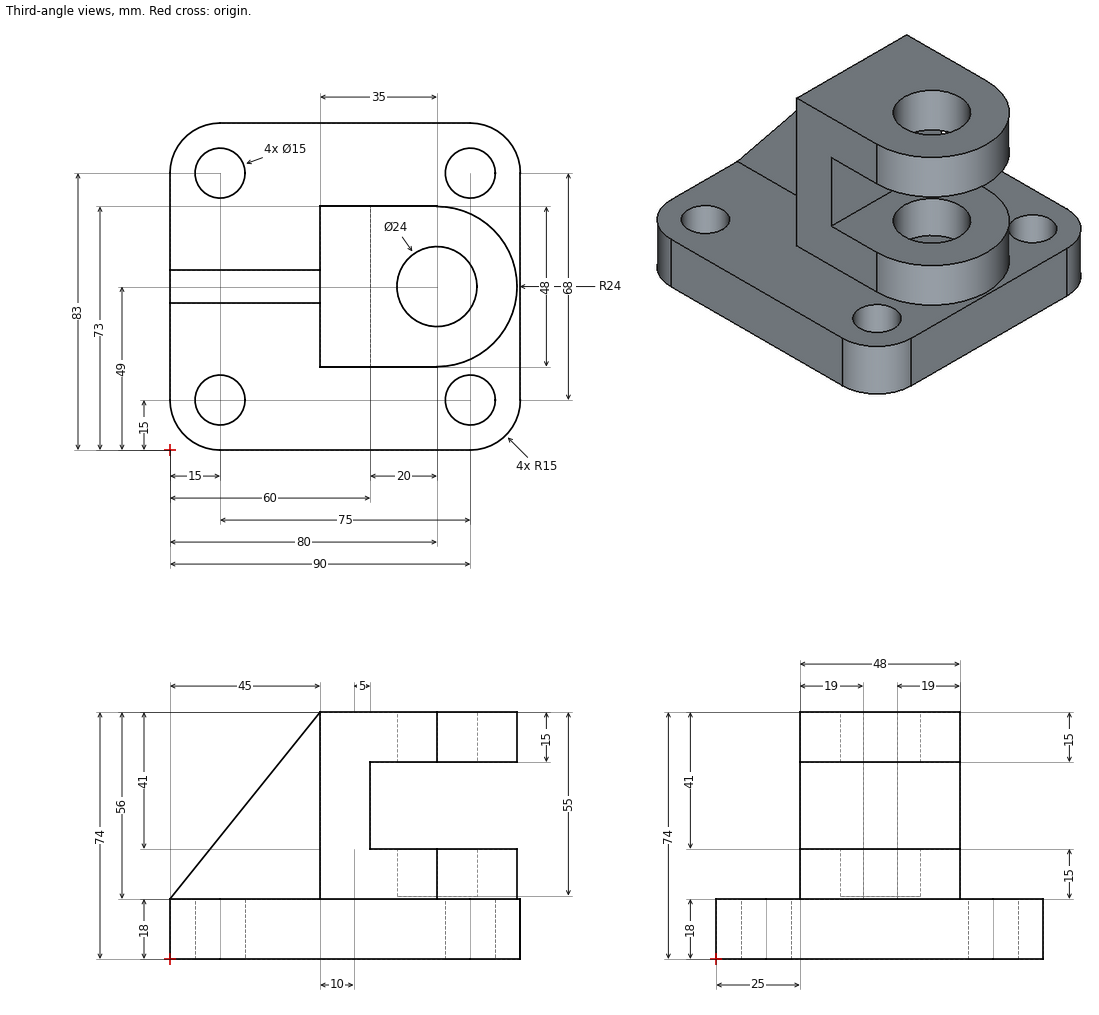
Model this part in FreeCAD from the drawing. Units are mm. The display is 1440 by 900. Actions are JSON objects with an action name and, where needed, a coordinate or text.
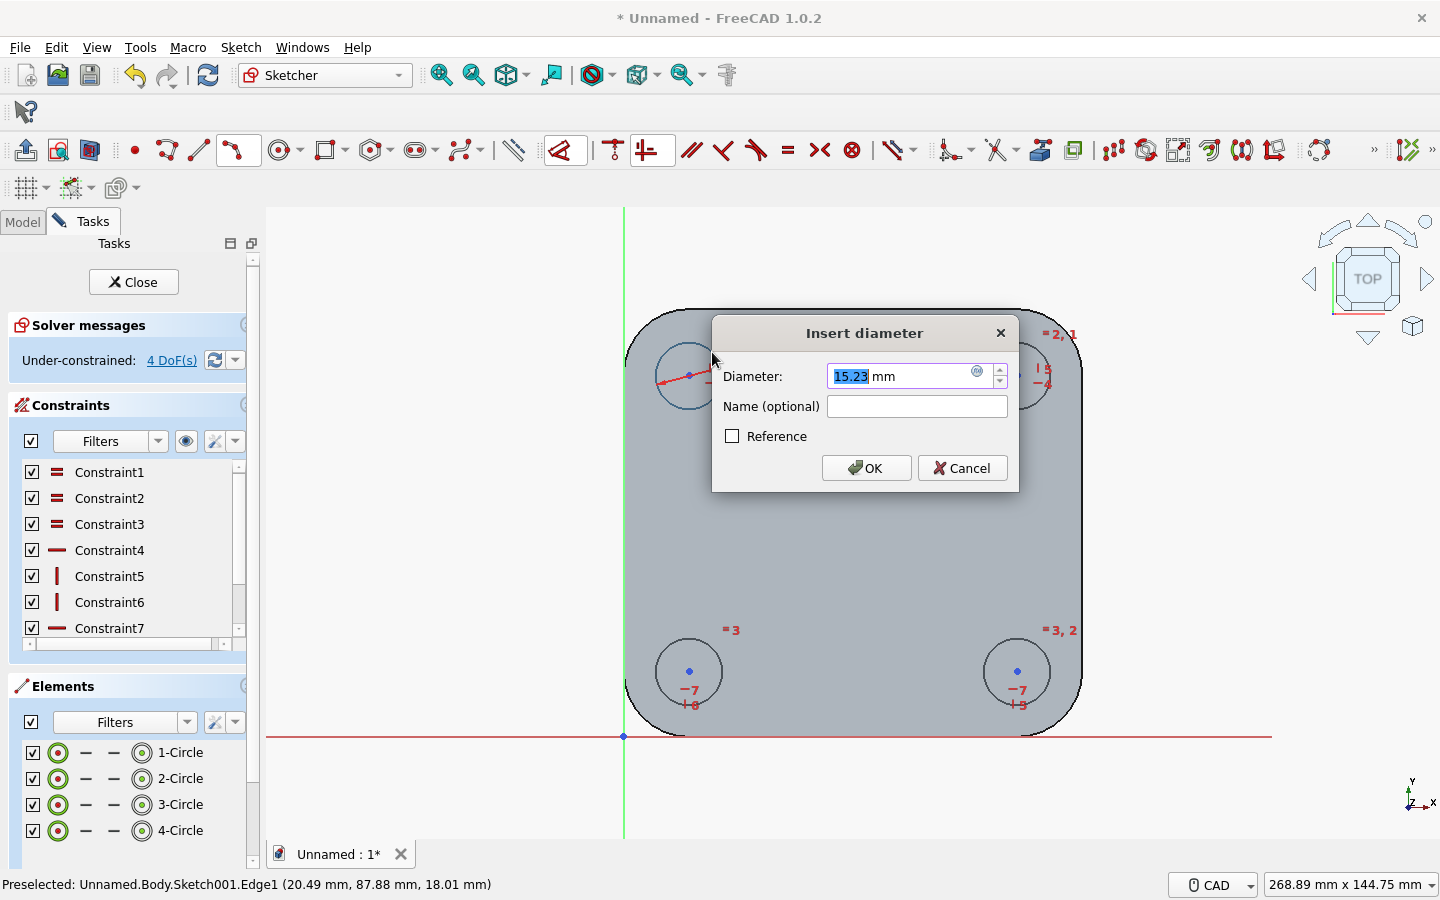
{"action": "type", "text": "15"}
{"action": "key", "text": "Return"}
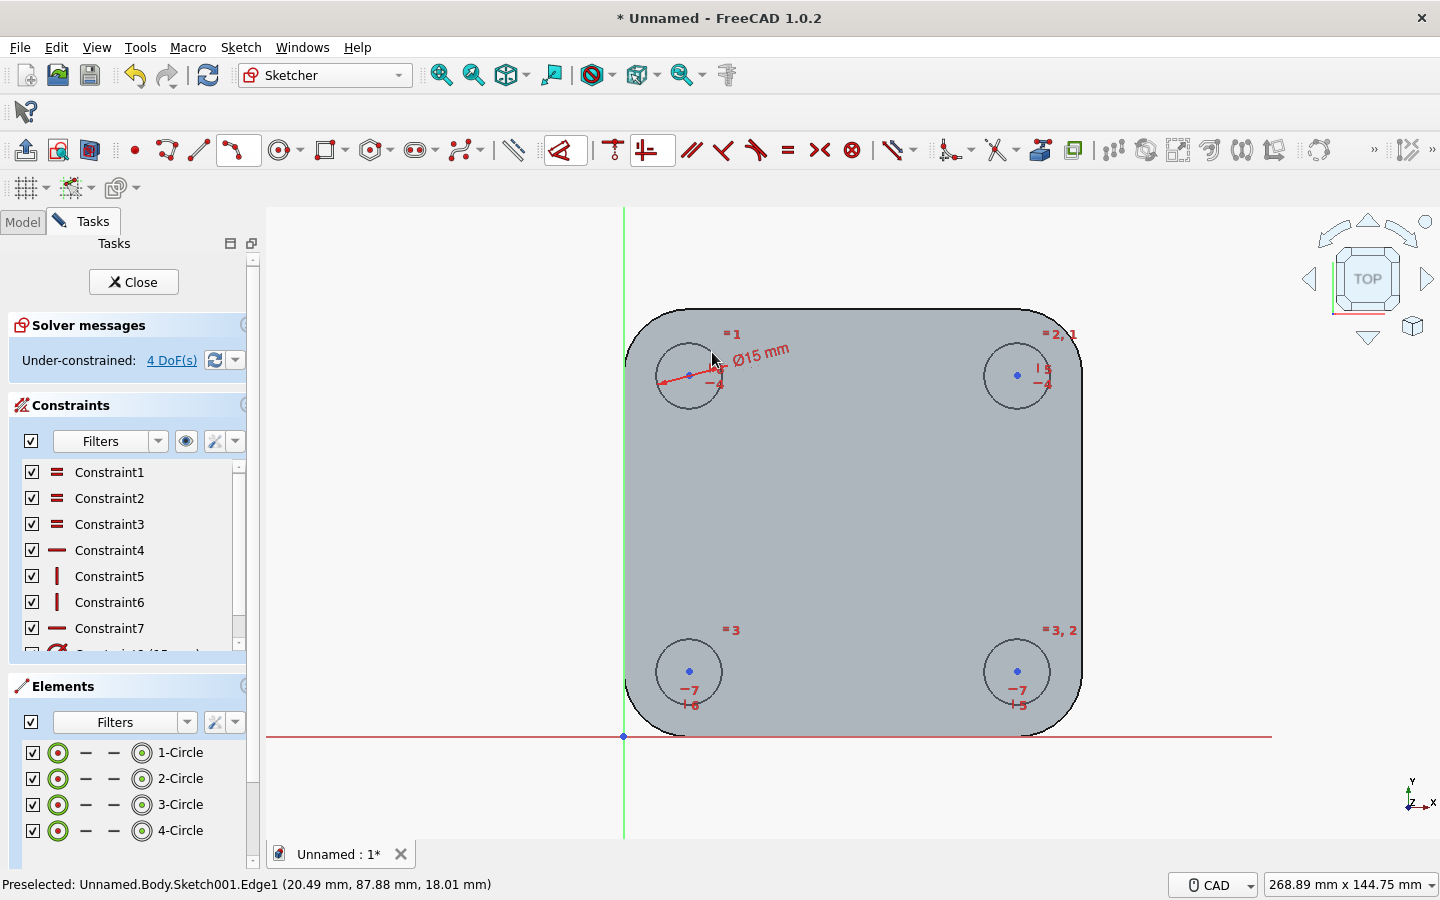
{"action": "left_click", "coordinate": [689, 376]}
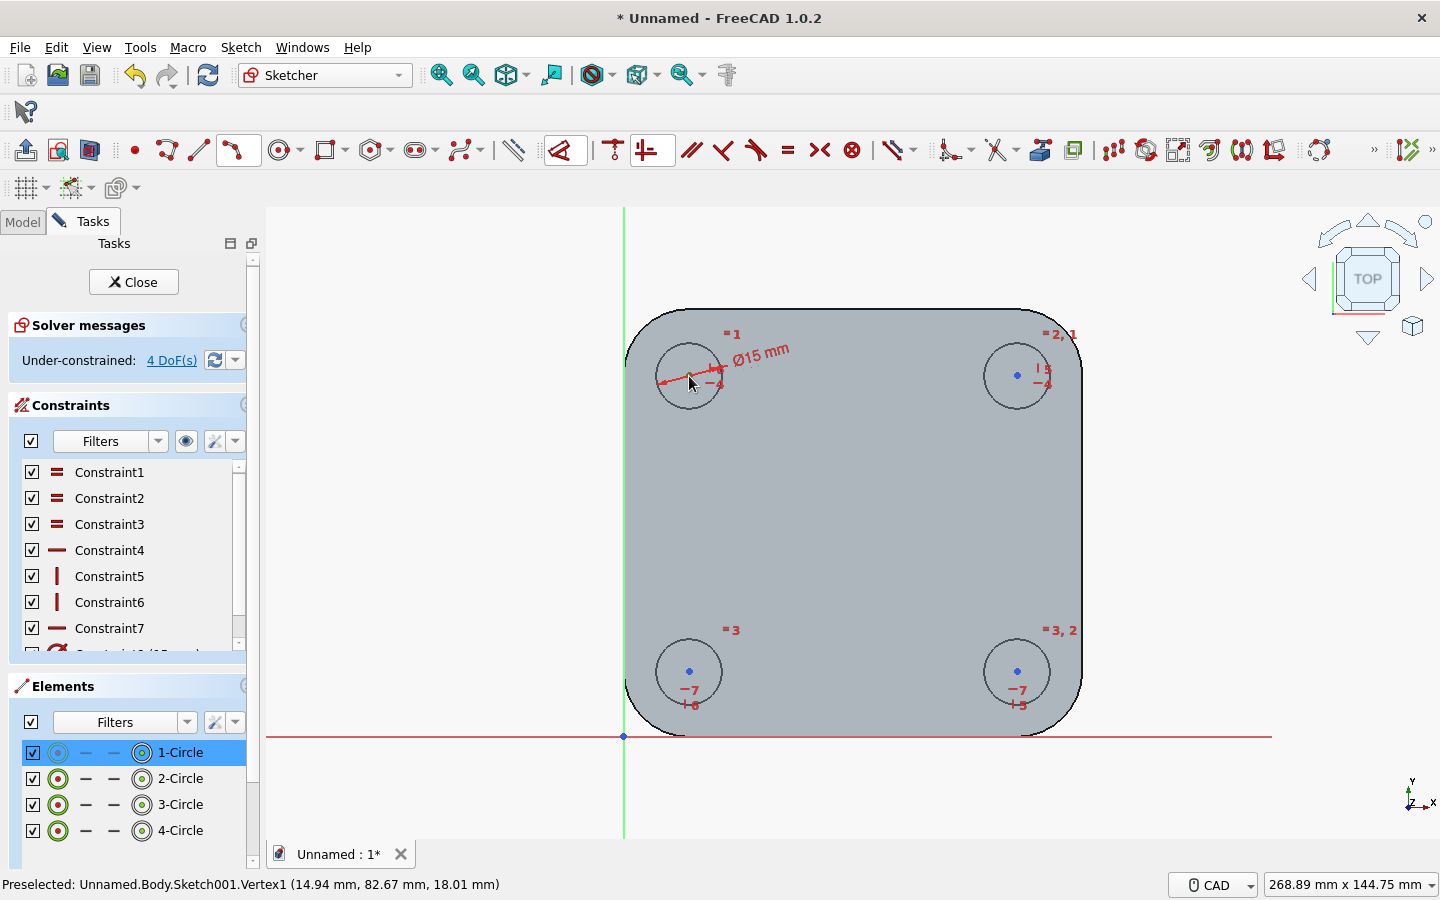
{"action": "key", "text": "l"}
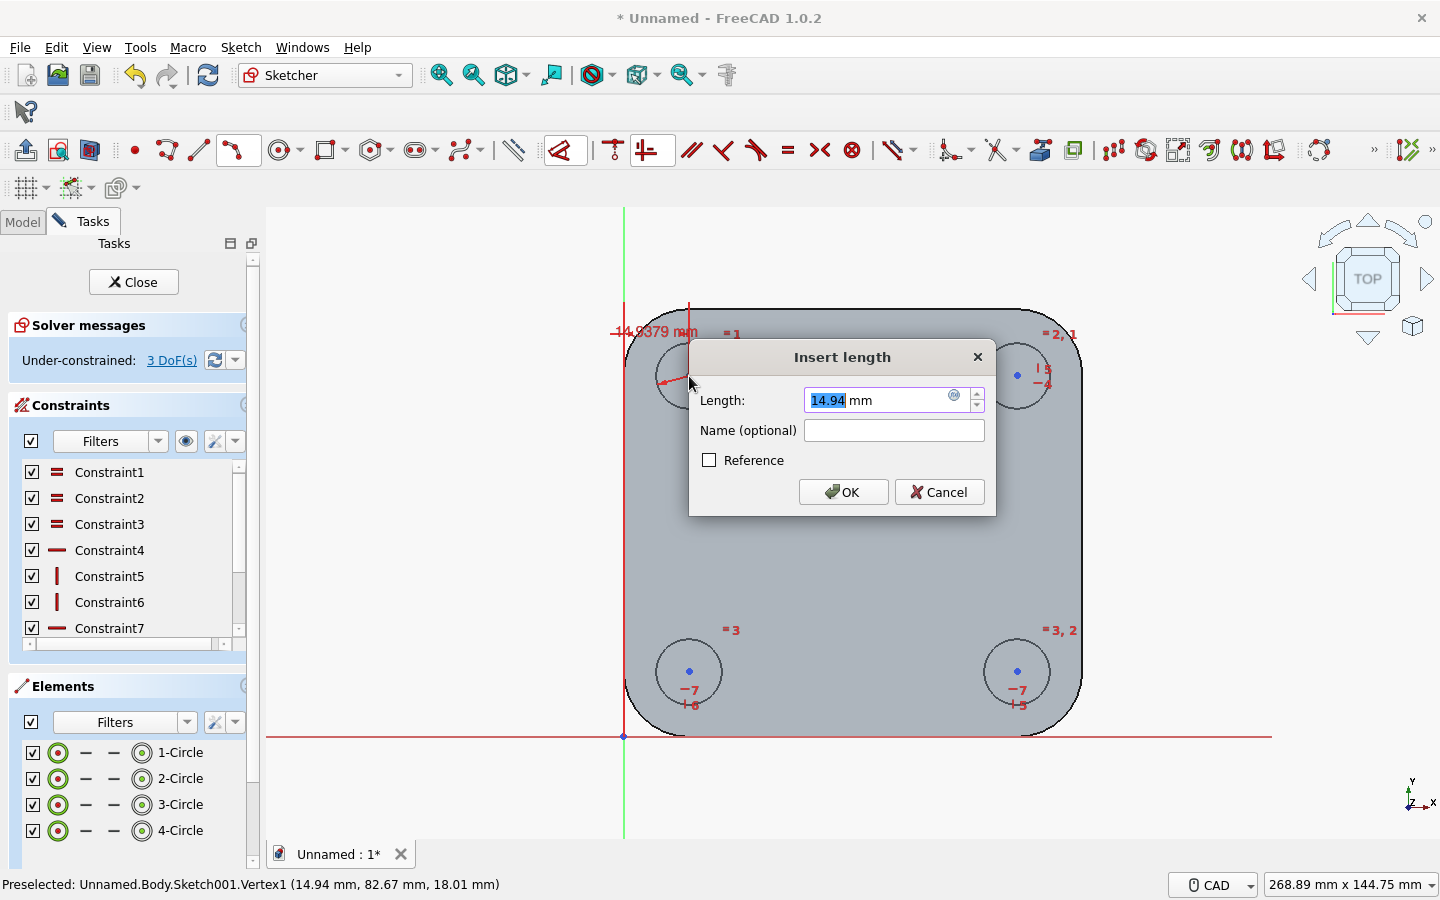
{"action": "type", "text": "15"}
{"action": "key", "text": "Return"}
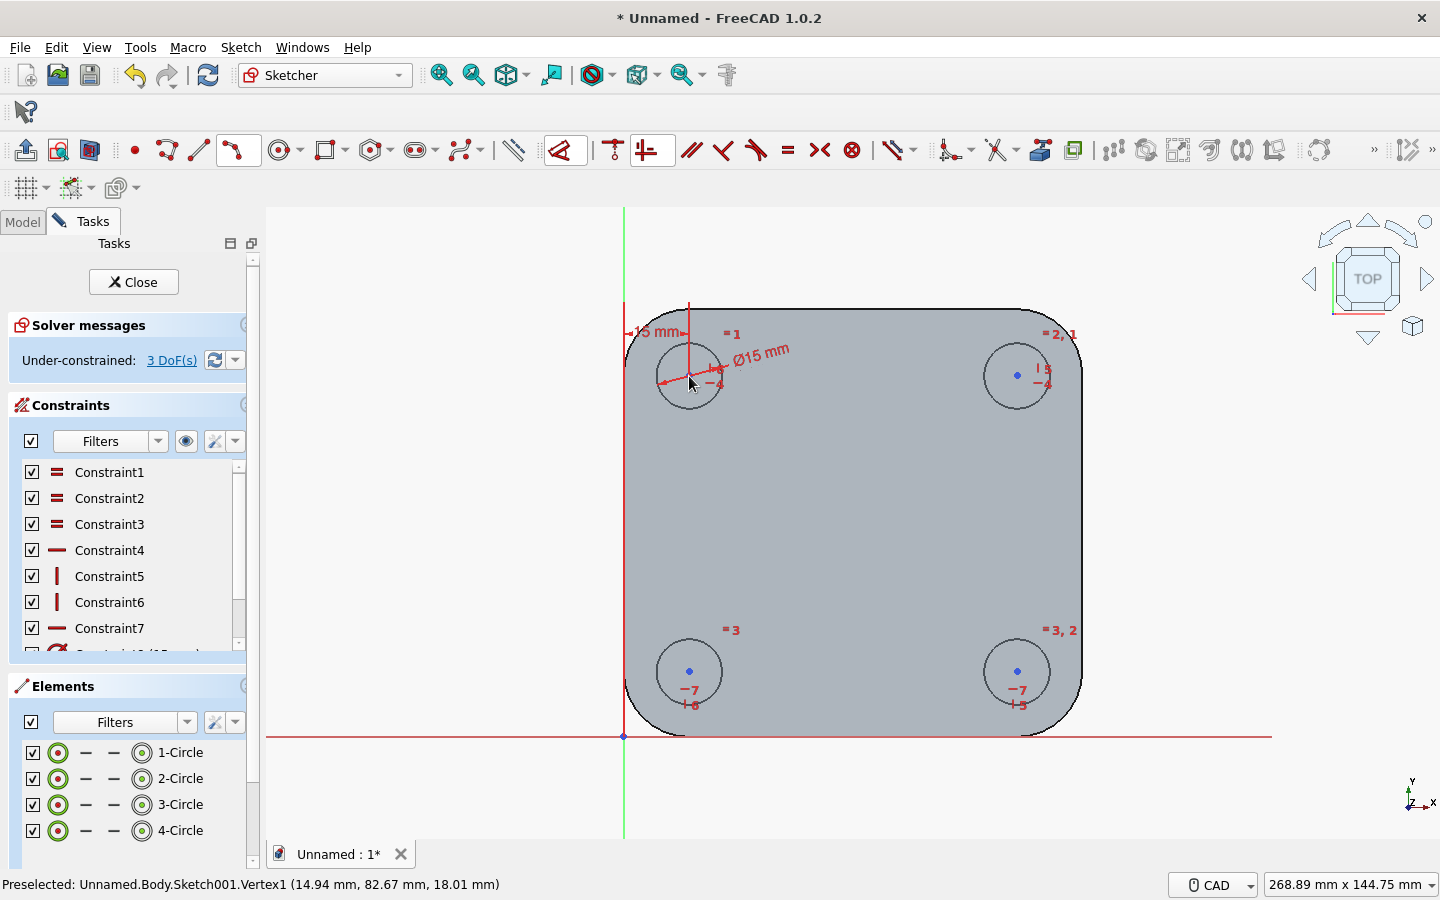
{"action": "left_click", "coordinate": [689, 376]}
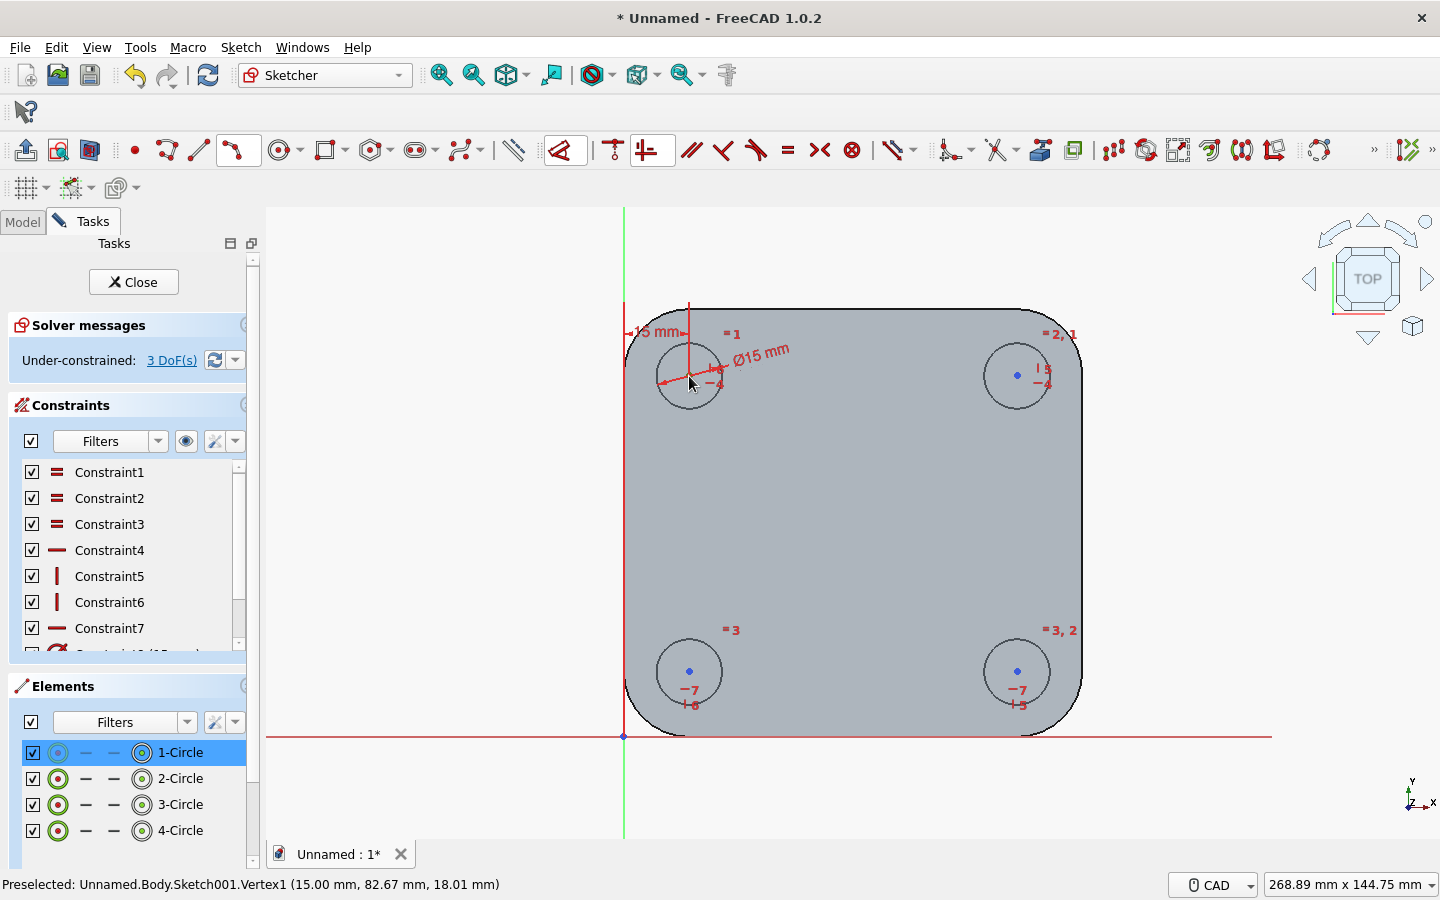
{"action": "key", "text": "i"}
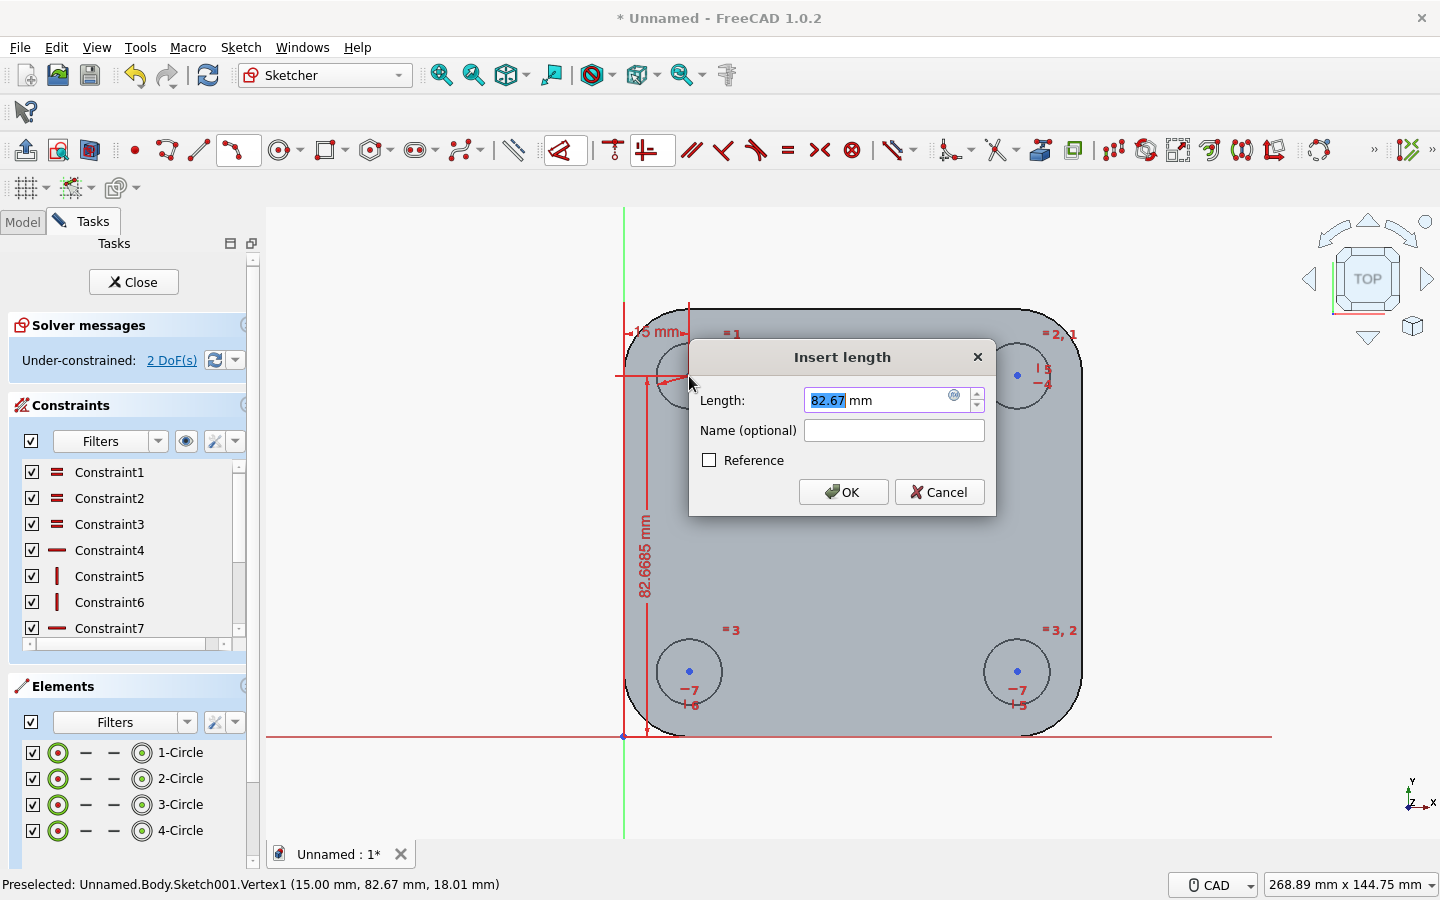
{"action": "type", "text": "83"}
{"action": "key", "text": "Return"}